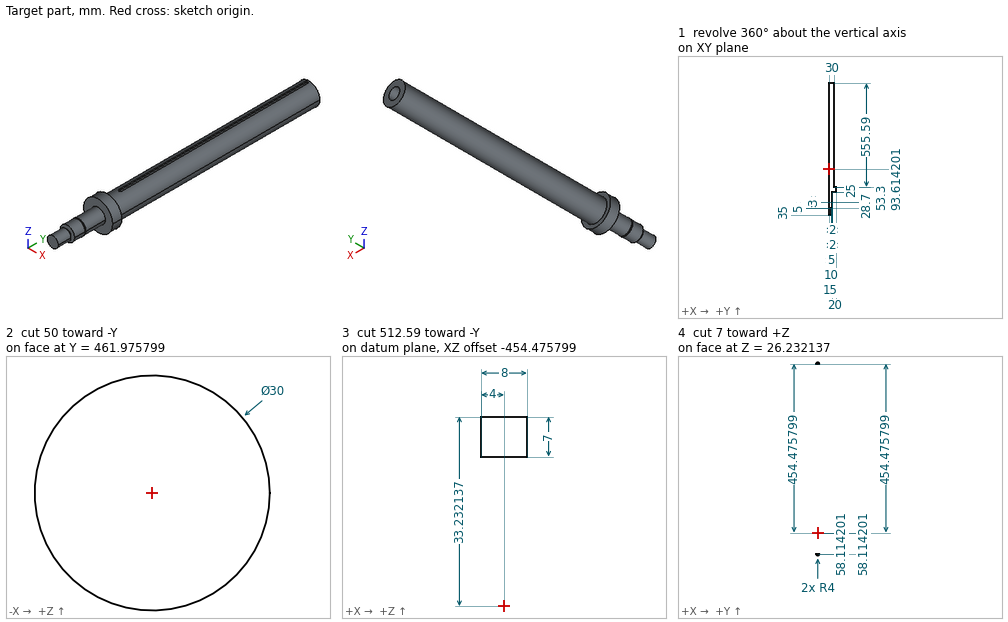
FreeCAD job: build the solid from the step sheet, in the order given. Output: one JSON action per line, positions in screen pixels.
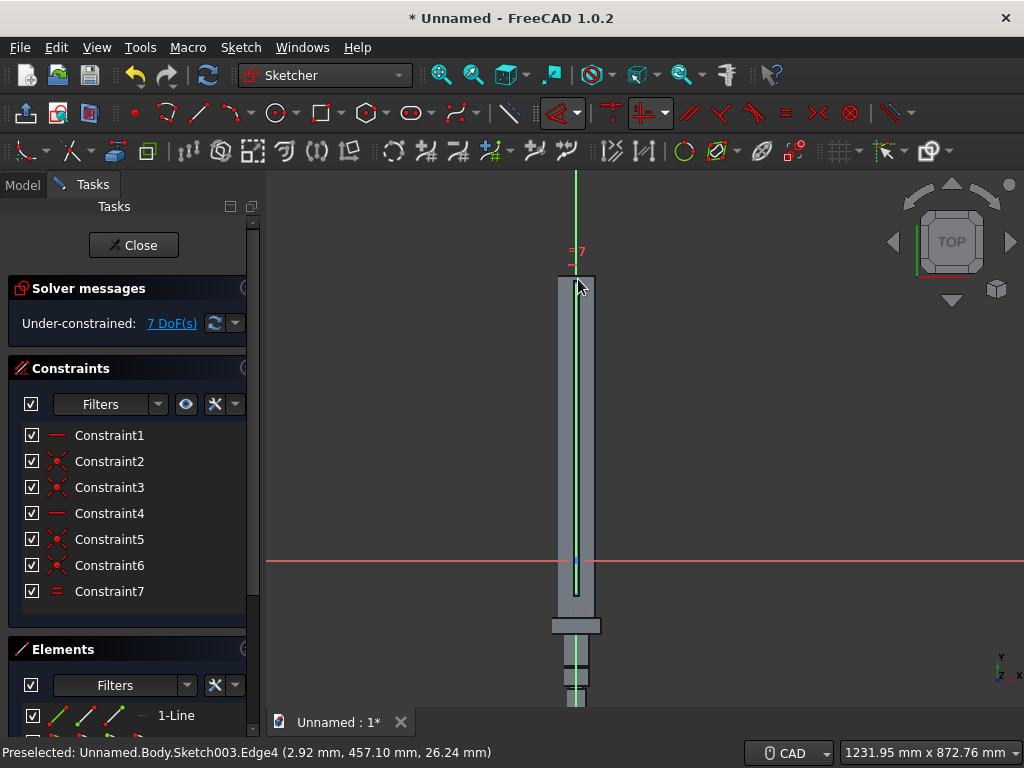
{"action": "scroll", "coordinate": [576, 596], "scroll_direction": "up", "scroll_amount": 9}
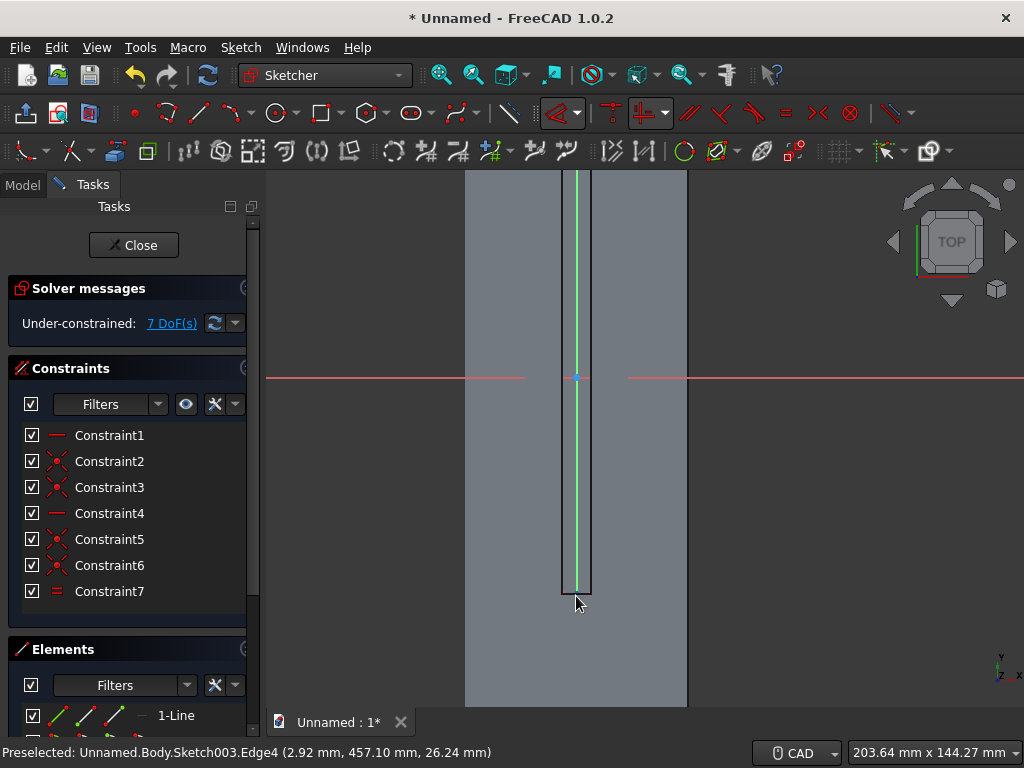
{"action": "left_click", "coordinate": [577, 595]}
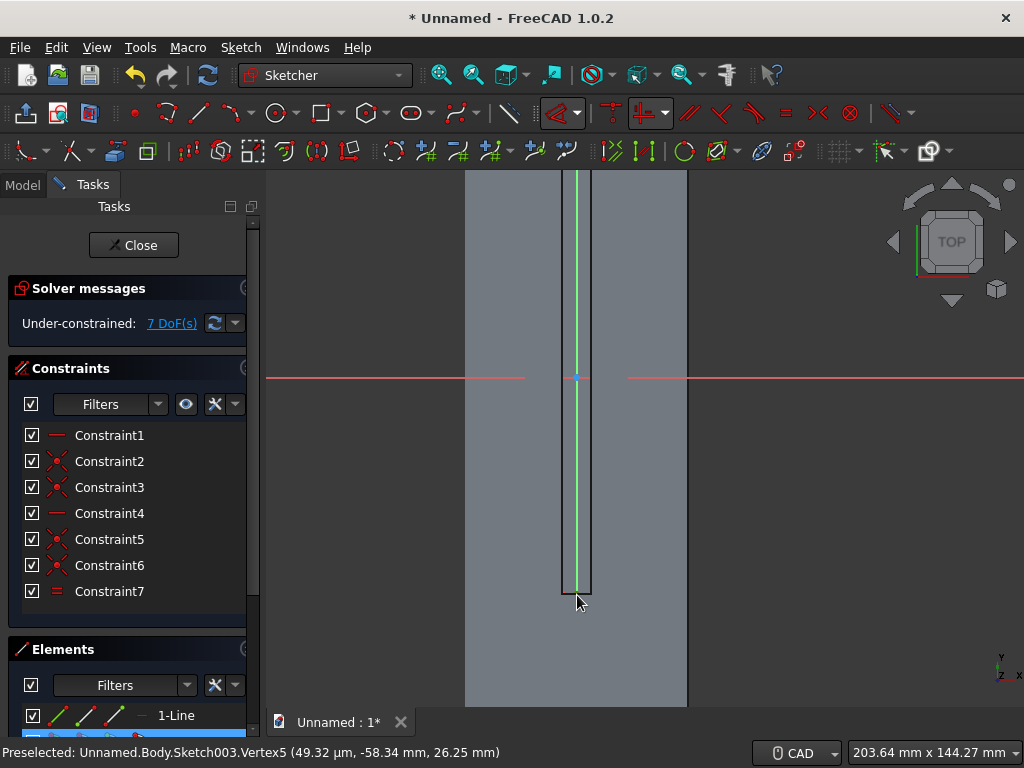
{"action": "left_click", "coordinate": [577, 645]}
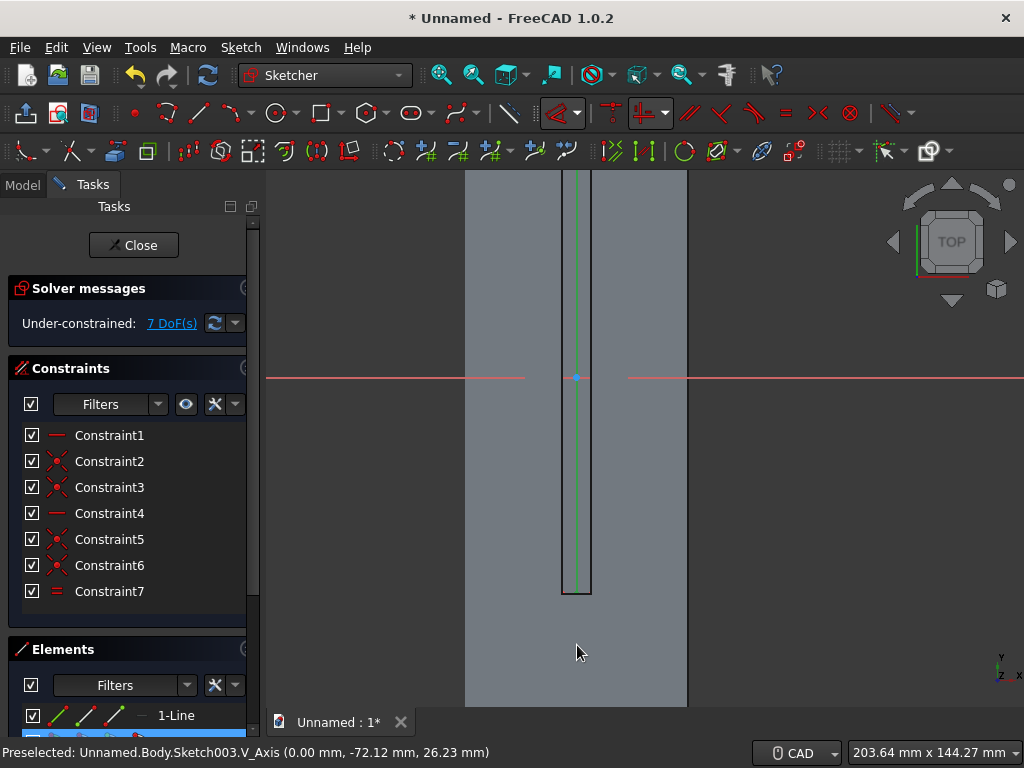
{"action": "key", "text": "c"}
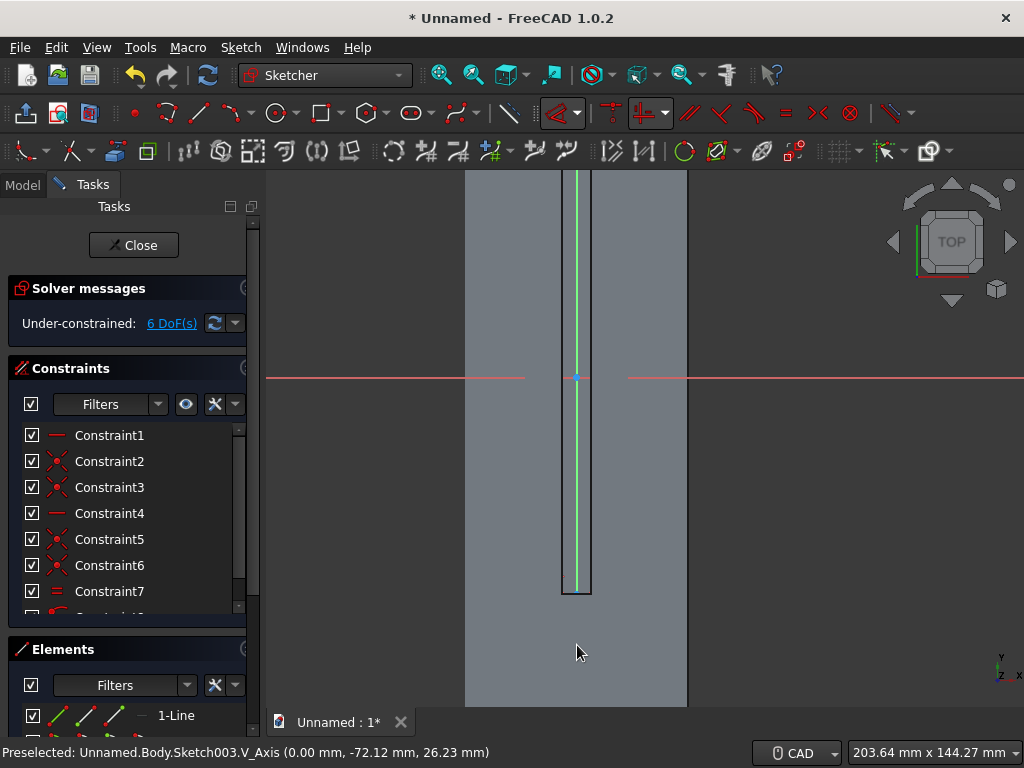
{"action": "scroll", "coordinate": [576, 597], "scroll_direction": "down", "scroll_amount": 9}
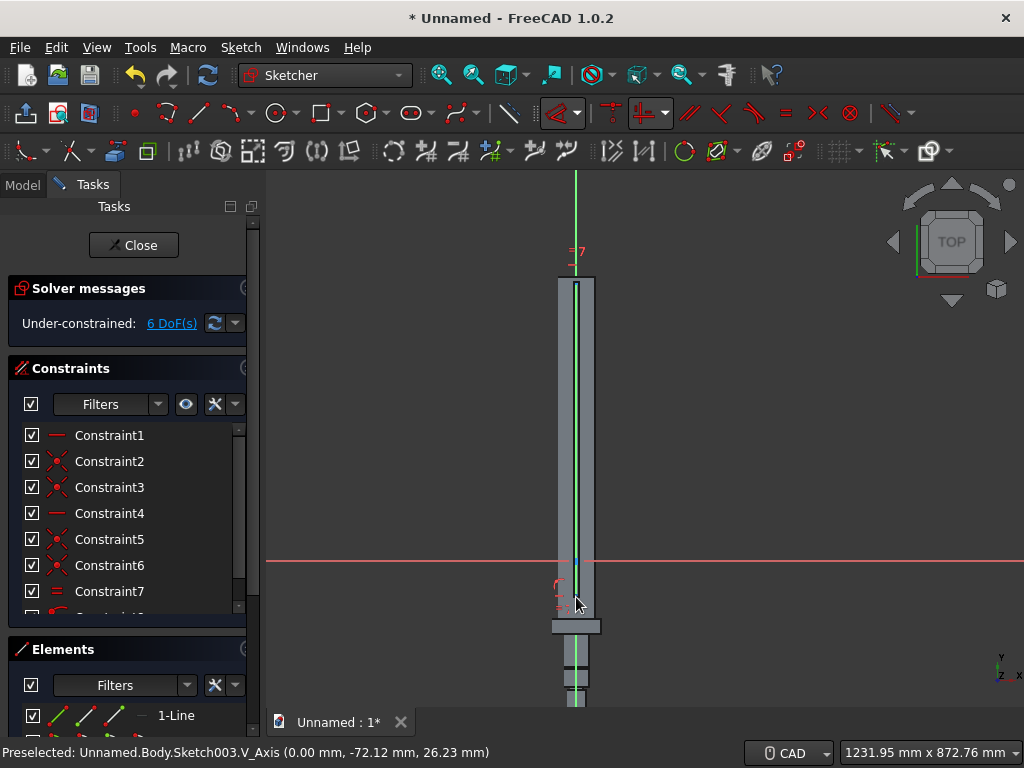
{"action": "scroll", "coordinate": [576, 282], "scroll_direction": "up", "scroll_amount": 9}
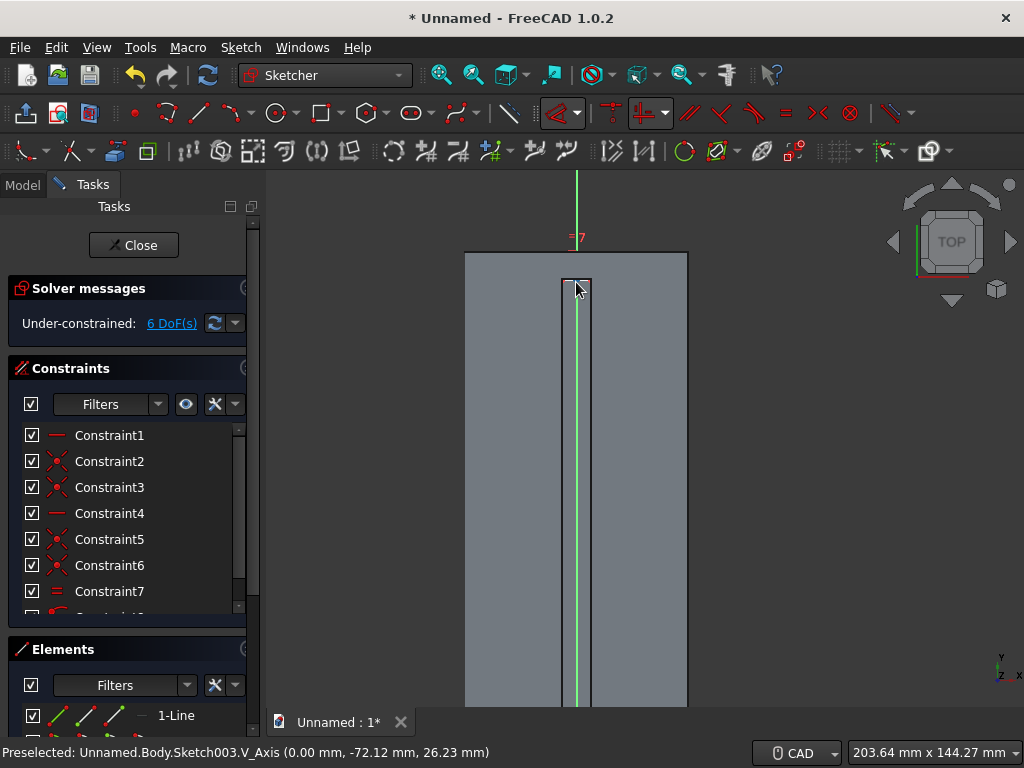
{"action": "left_click", "coordinate": [576, 280]}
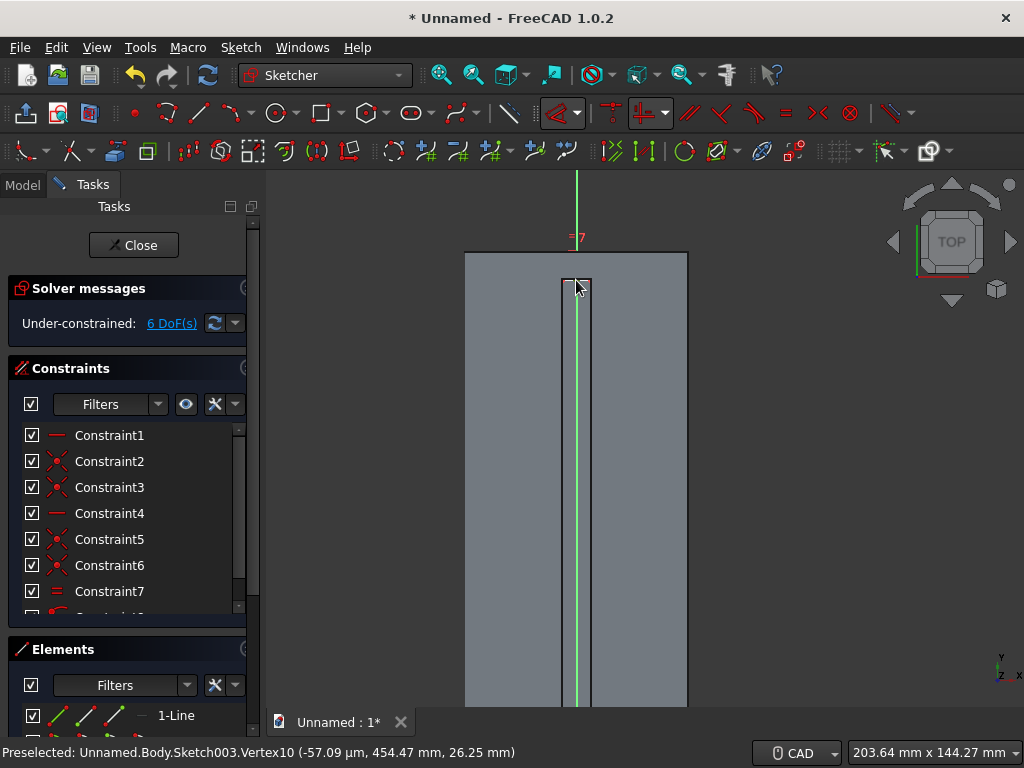
{"action": "left_click", "coordinate": [577, 645]}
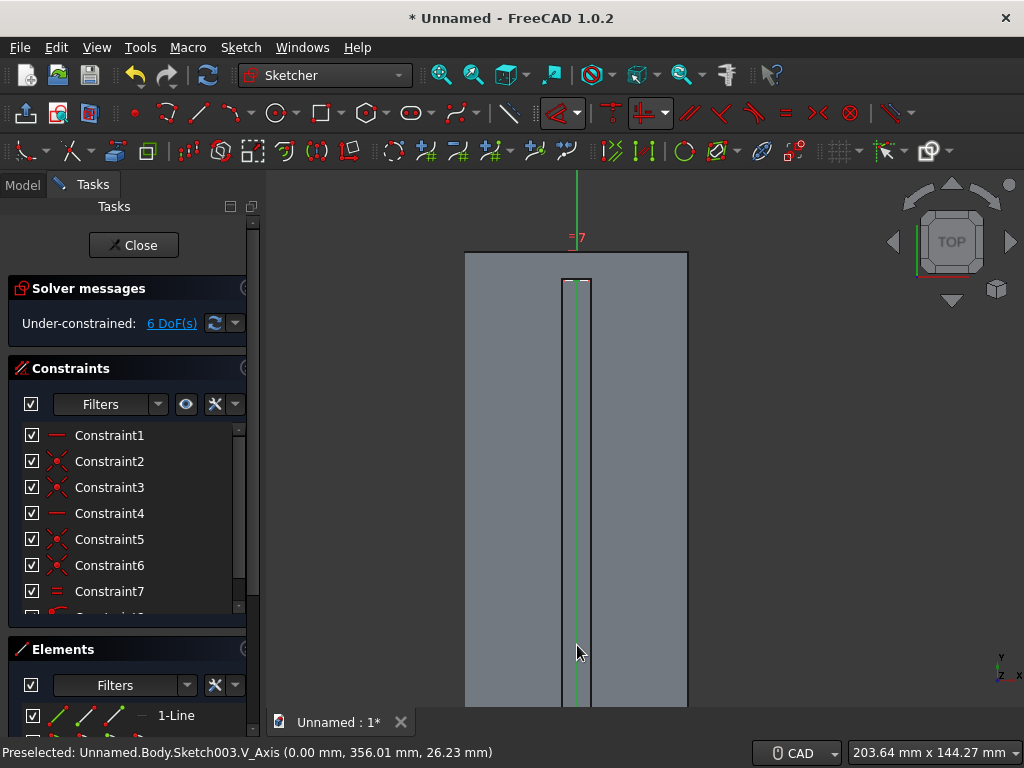
{"action": "key", "text": "c"}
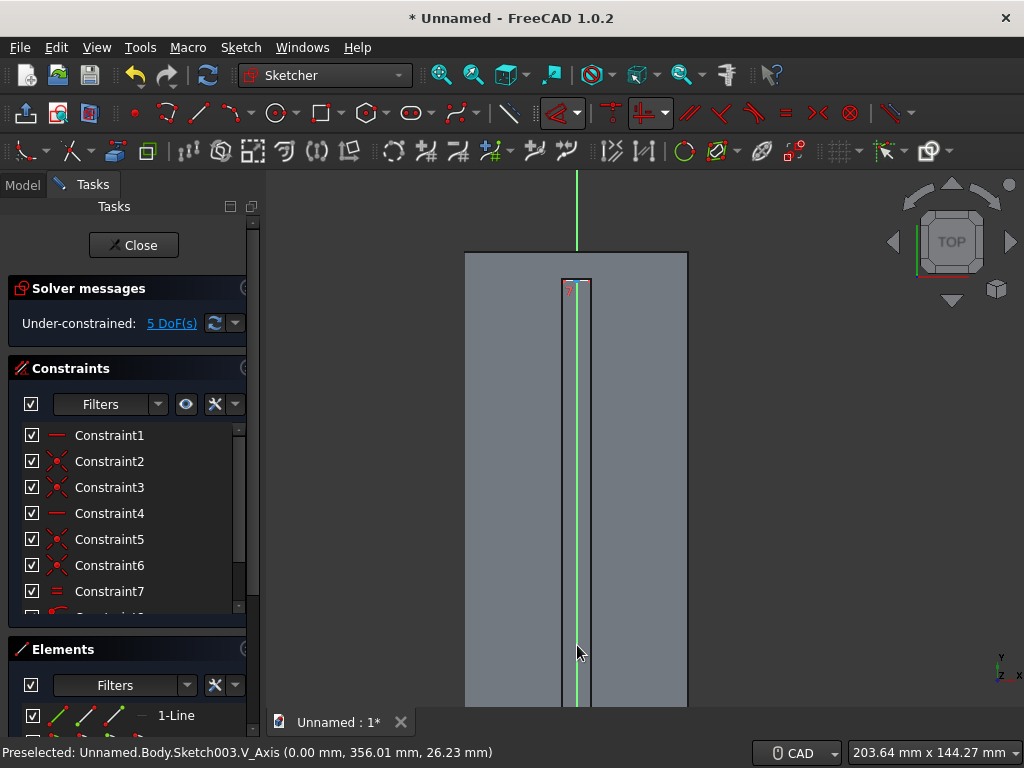
{"action": "left_click", "coordinate": [556, 114]}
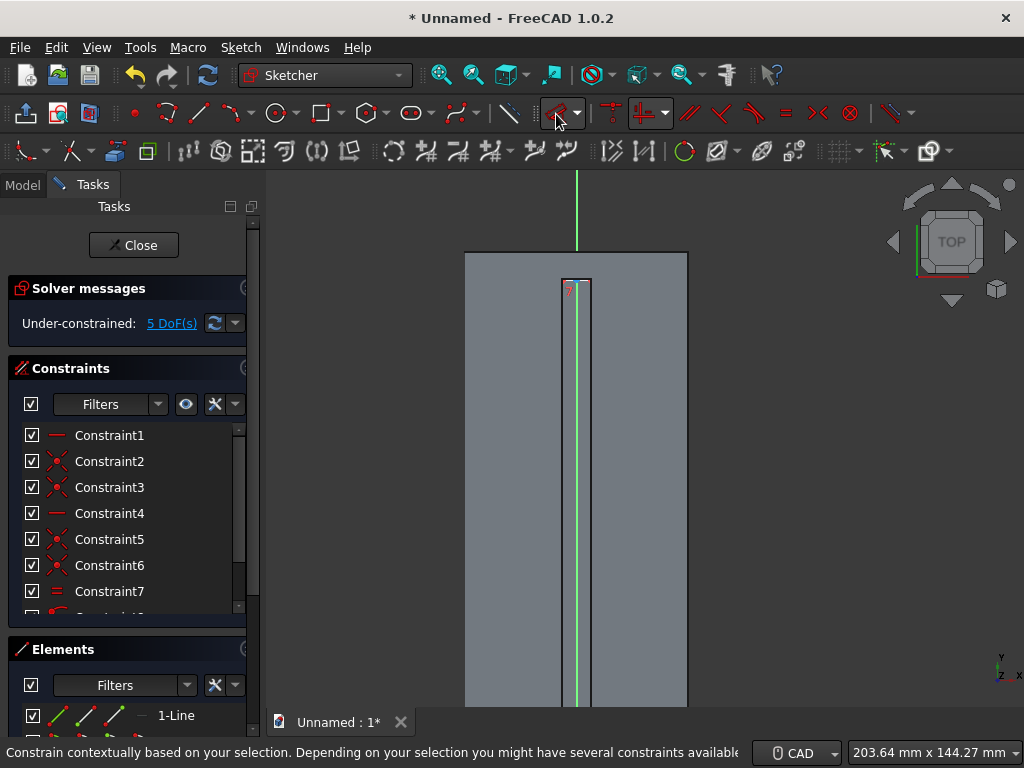
{"action": "scroll", "coordinate": [576, 281], "scroll_direction": "down", "scroll_amount": 9}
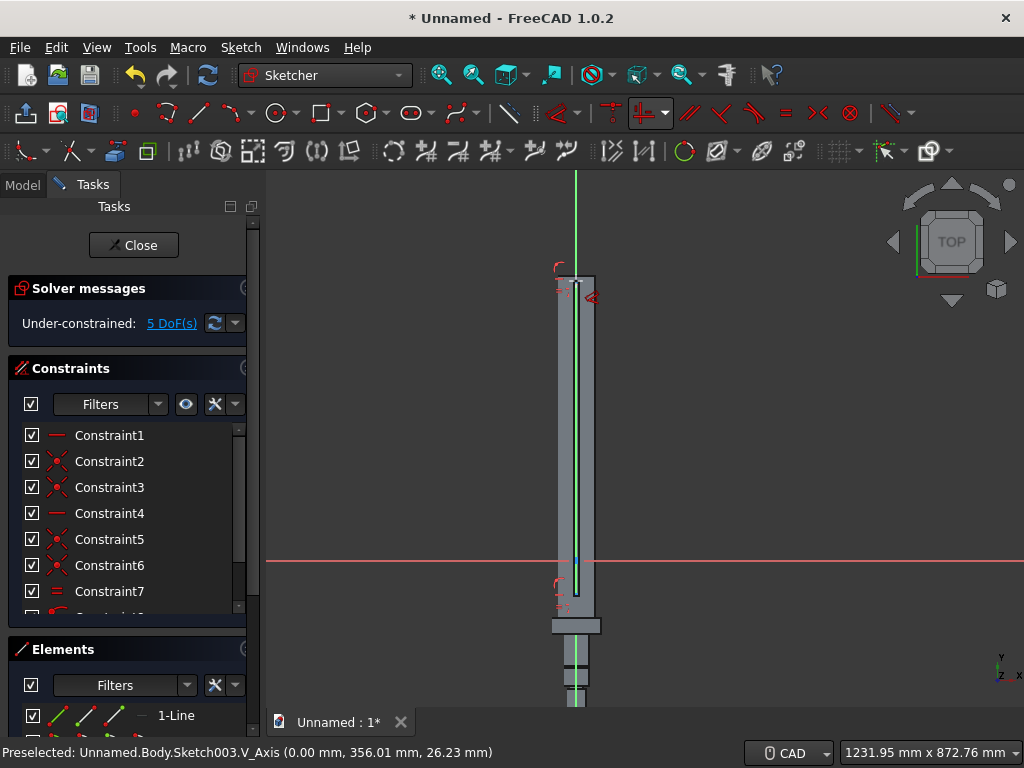
{"action": "scroll", "coordinate": [576, 599], "scroll_direction": "up", "scroll_amount": 14}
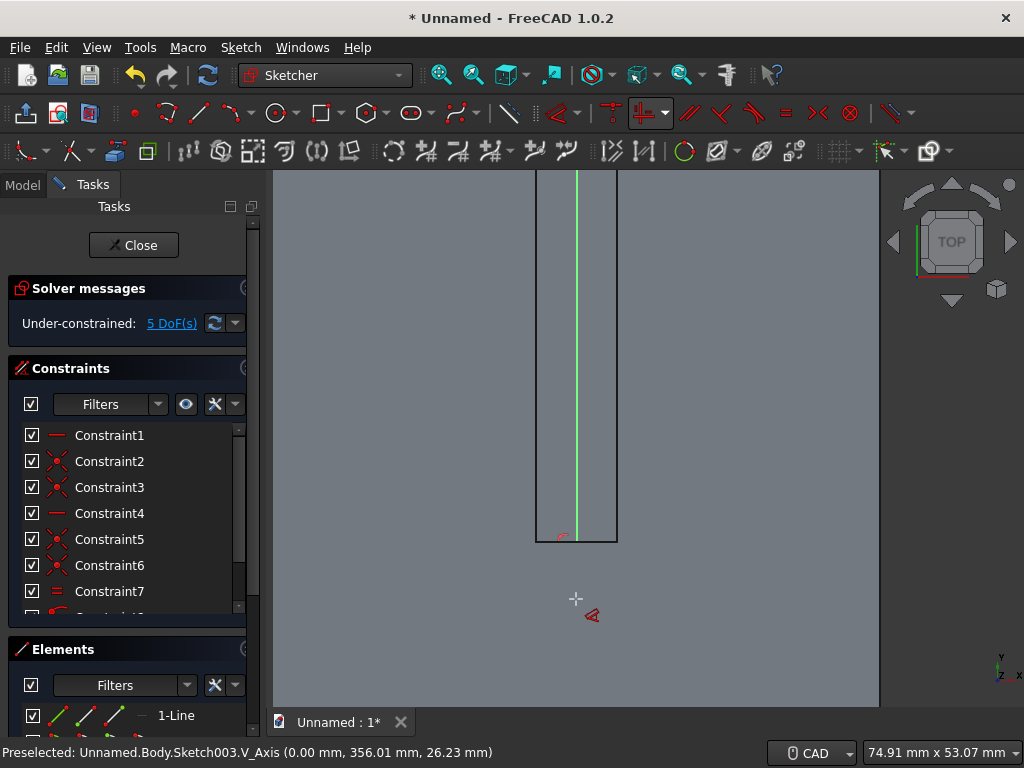
{"action": "left_click", "coordinate": [577, 584]}
{"action": "left_click", "coordinate": [543, 607]}